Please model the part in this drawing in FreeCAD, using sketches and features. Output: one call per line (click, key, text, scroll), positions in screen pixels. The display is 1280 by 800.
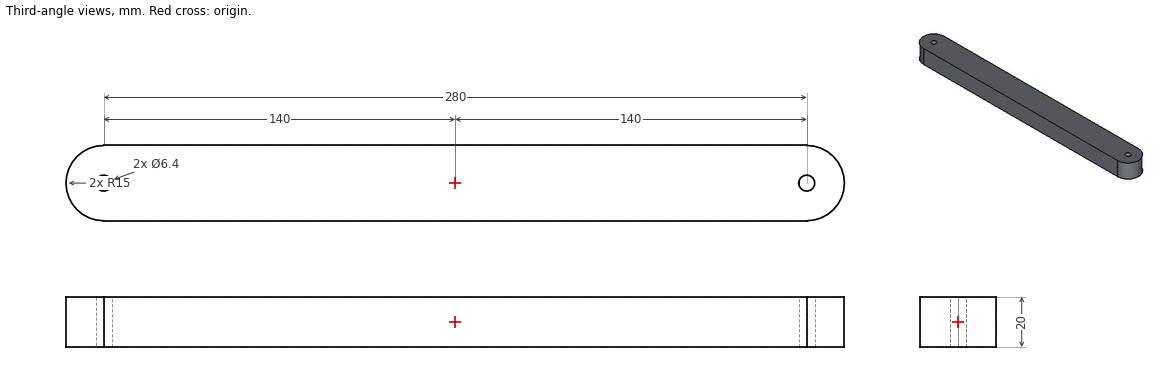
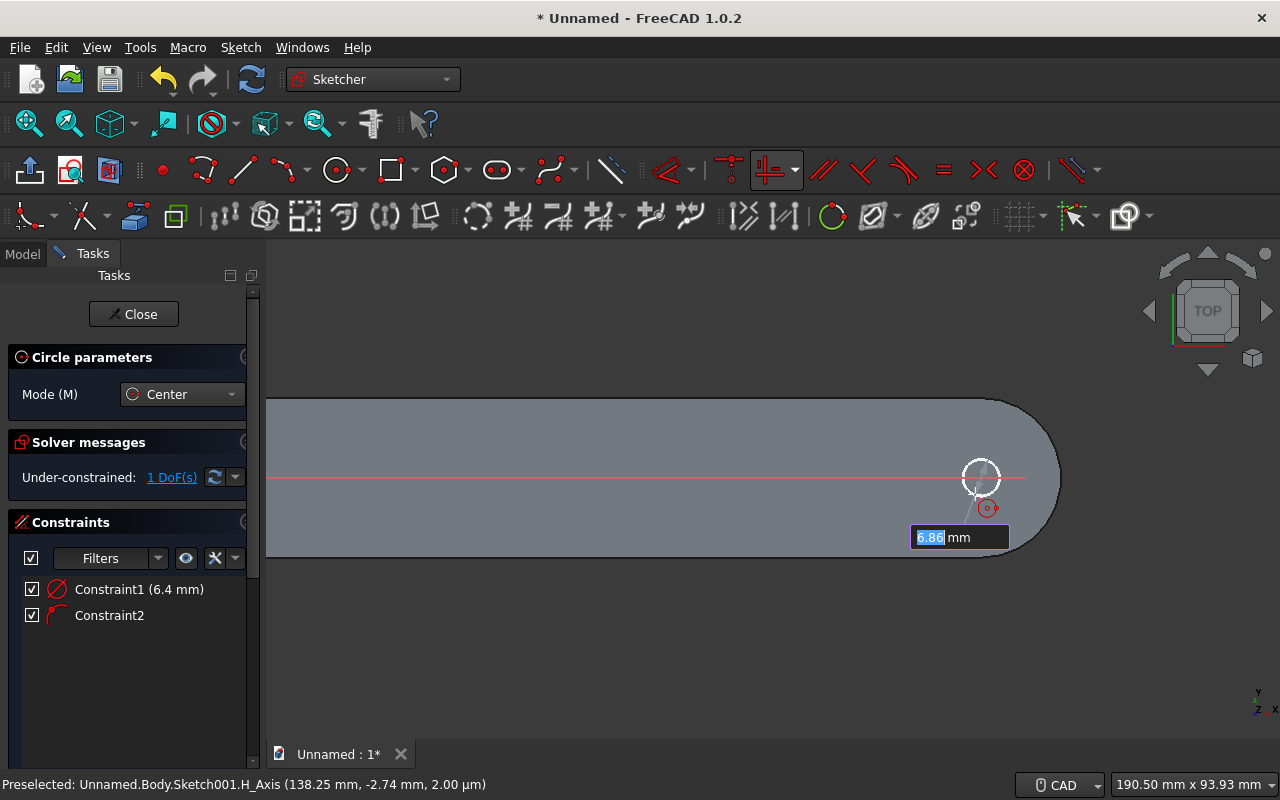
text(6.4)
key(Return)
key(Escape)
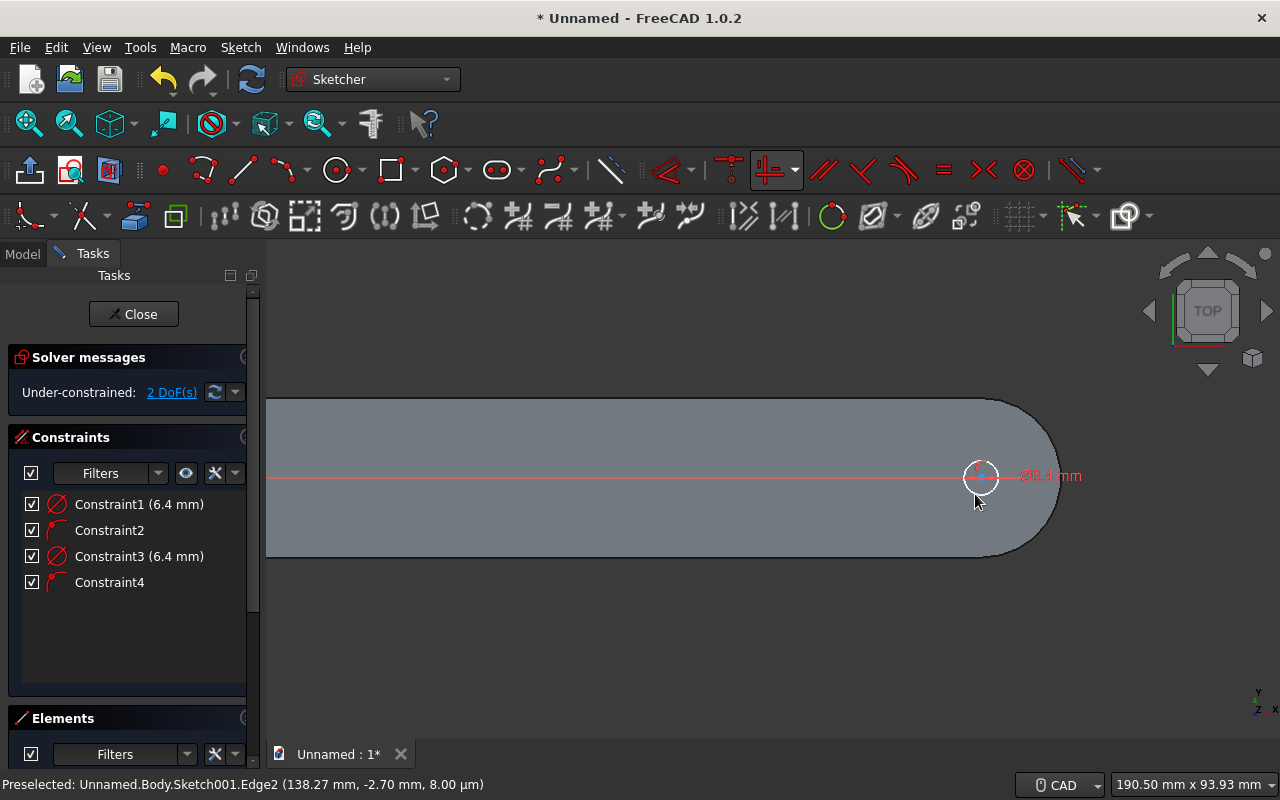
scroll(977, 495, down, 5)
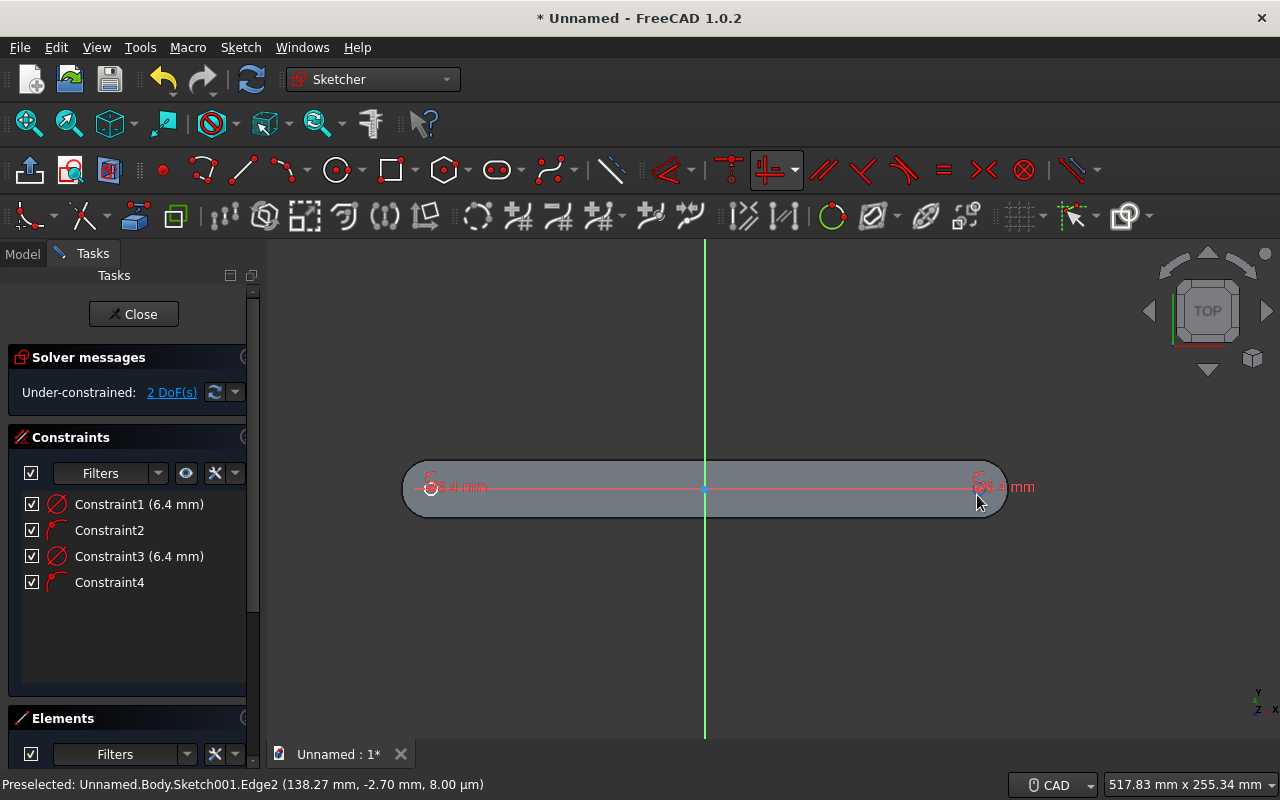
click(431, 489)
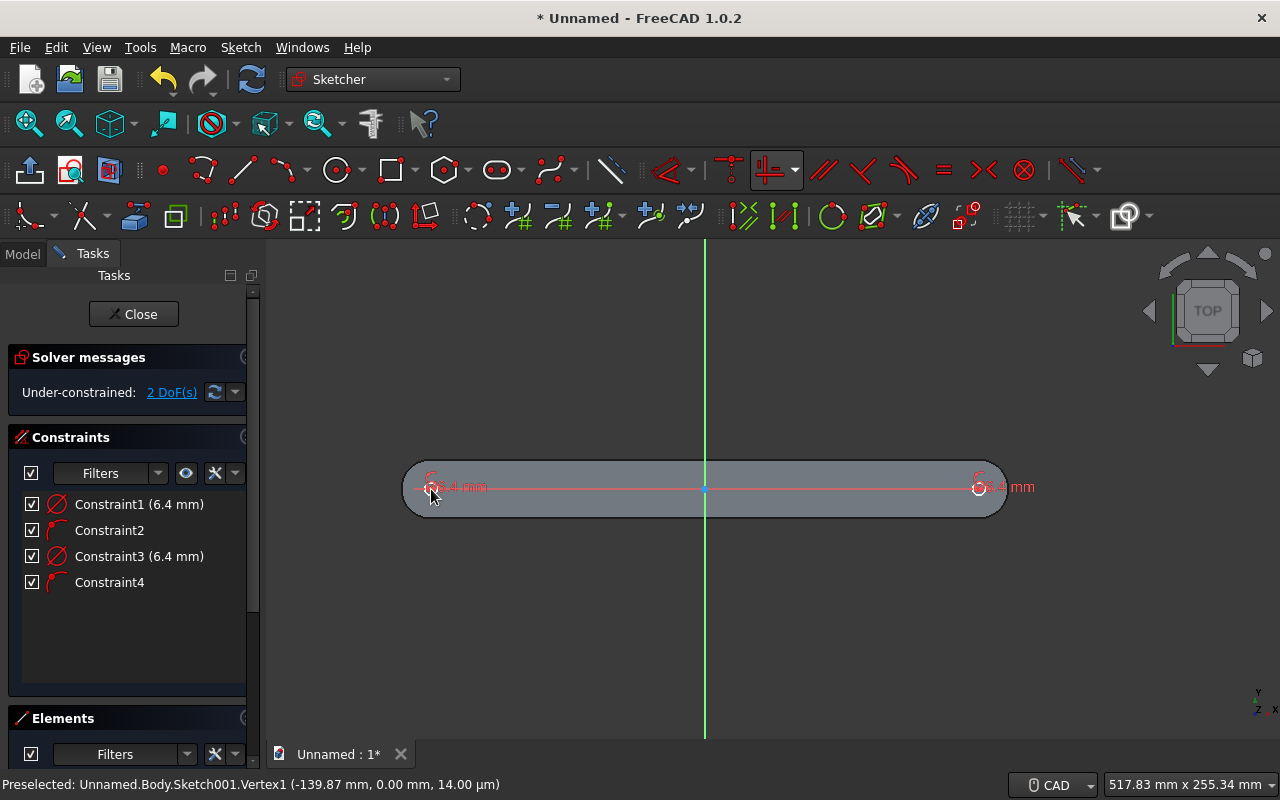
click(694, 170)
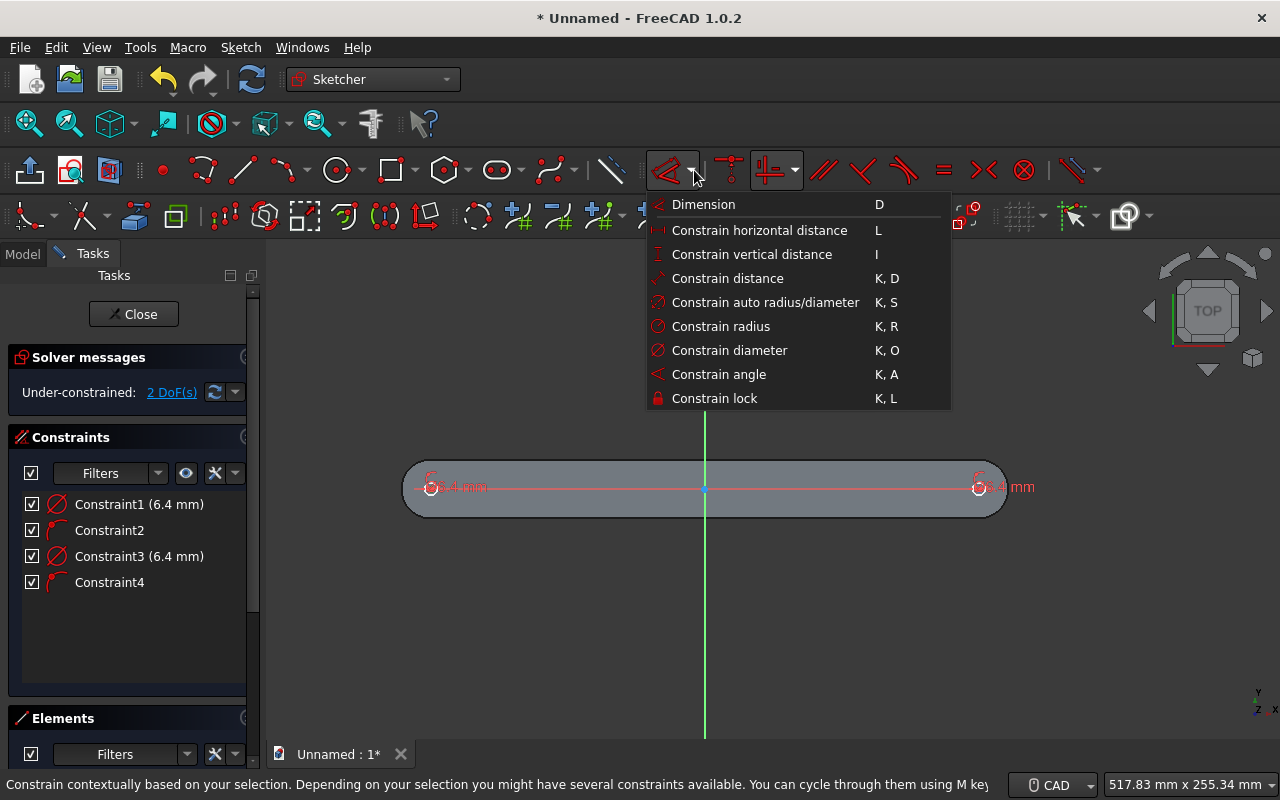
click(799, 230)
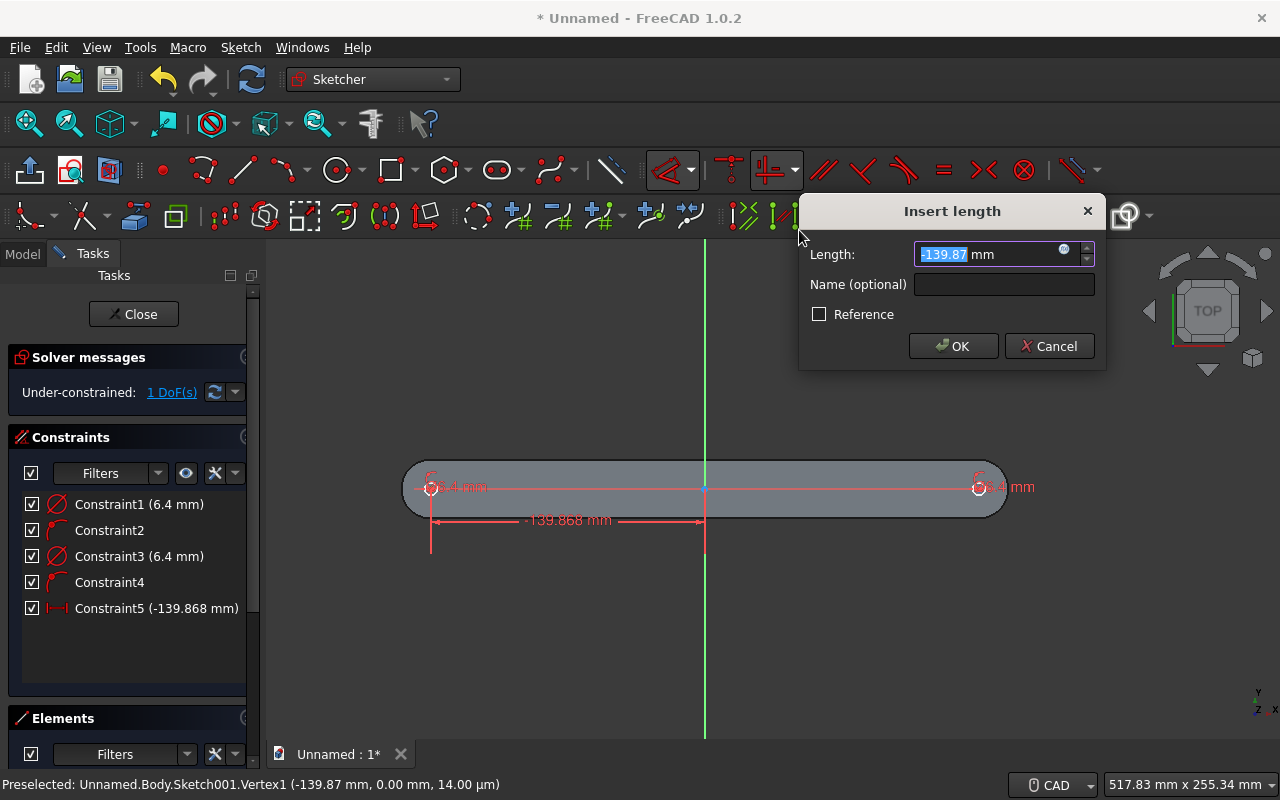
text(-140)
key(Return)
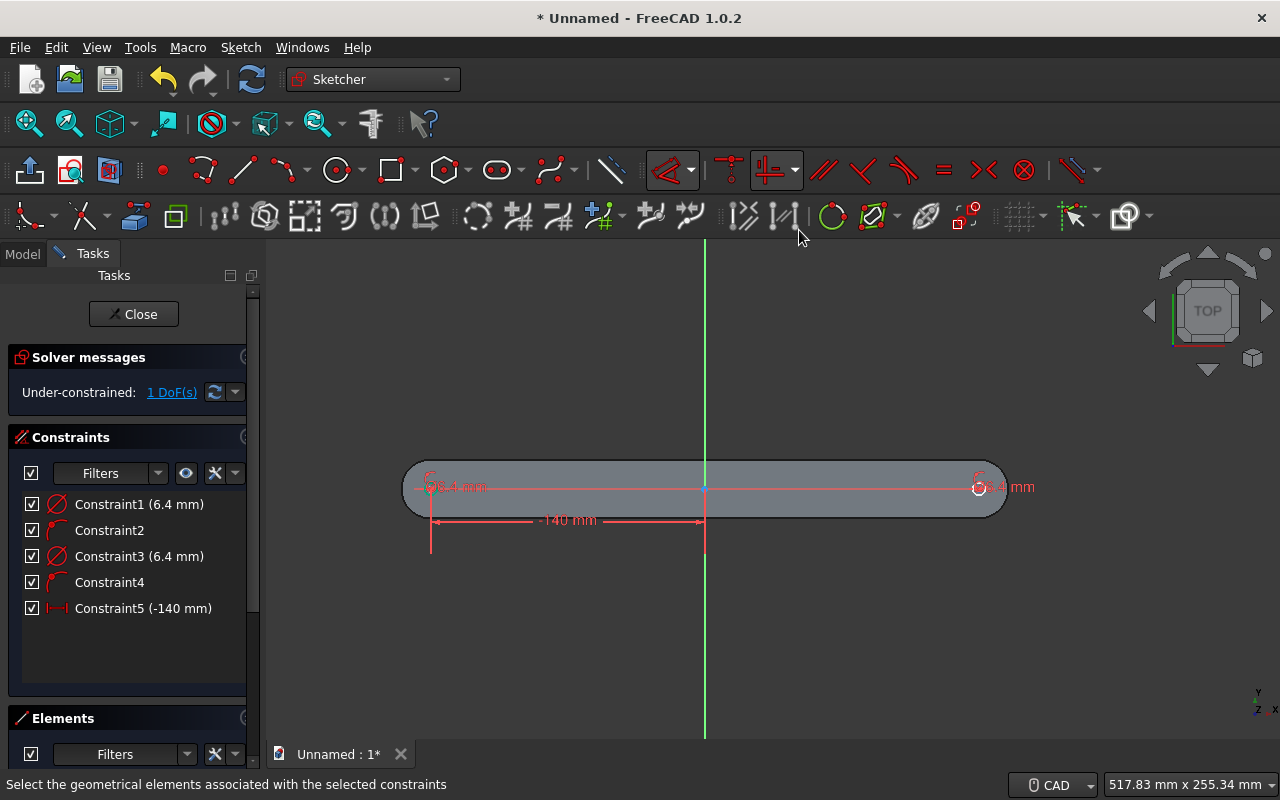
click(979, 489)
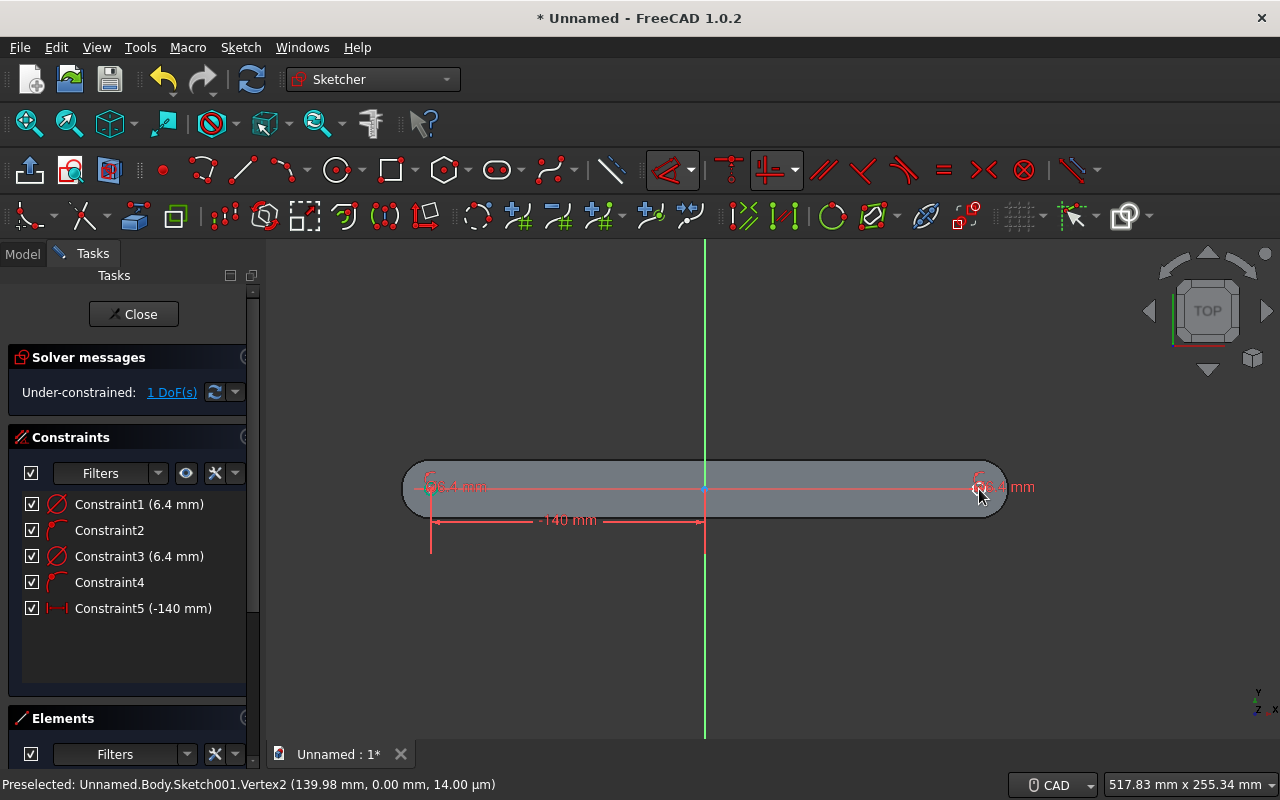
click(694, 170)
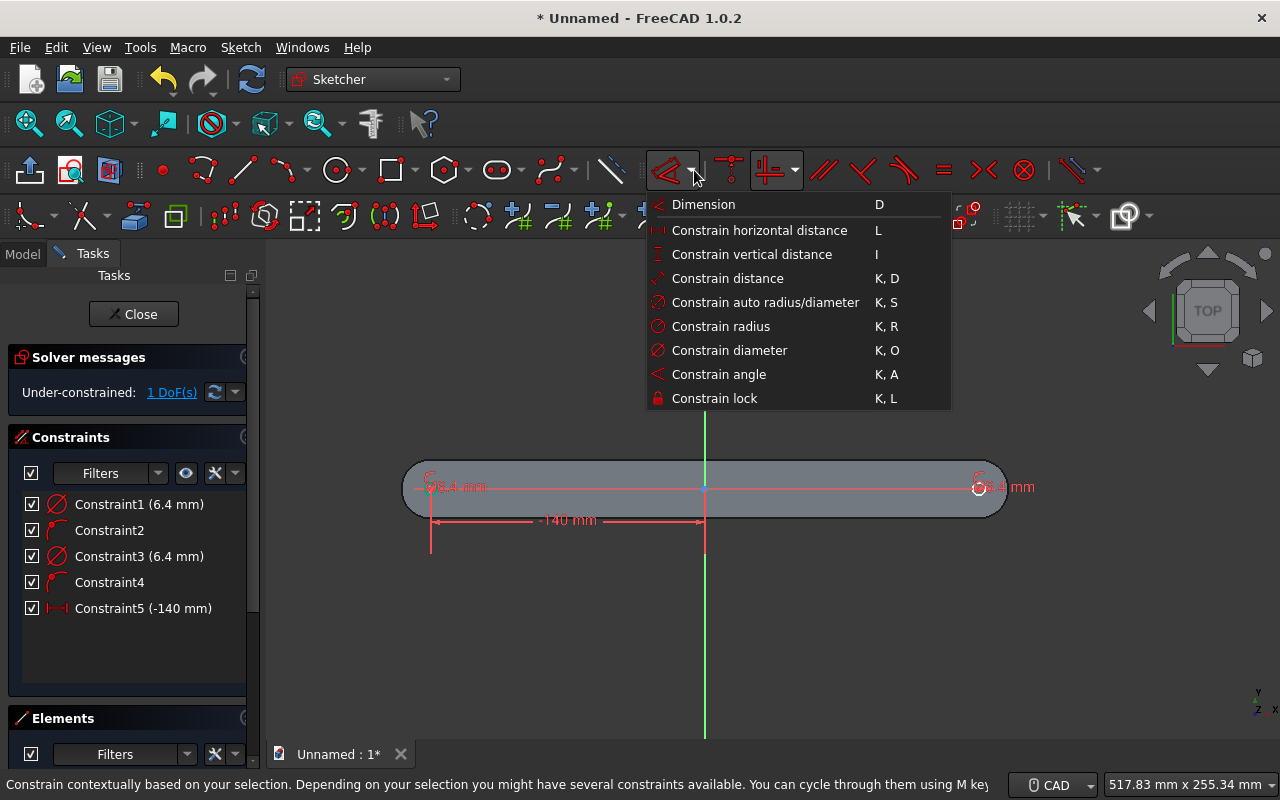
click(799, 230)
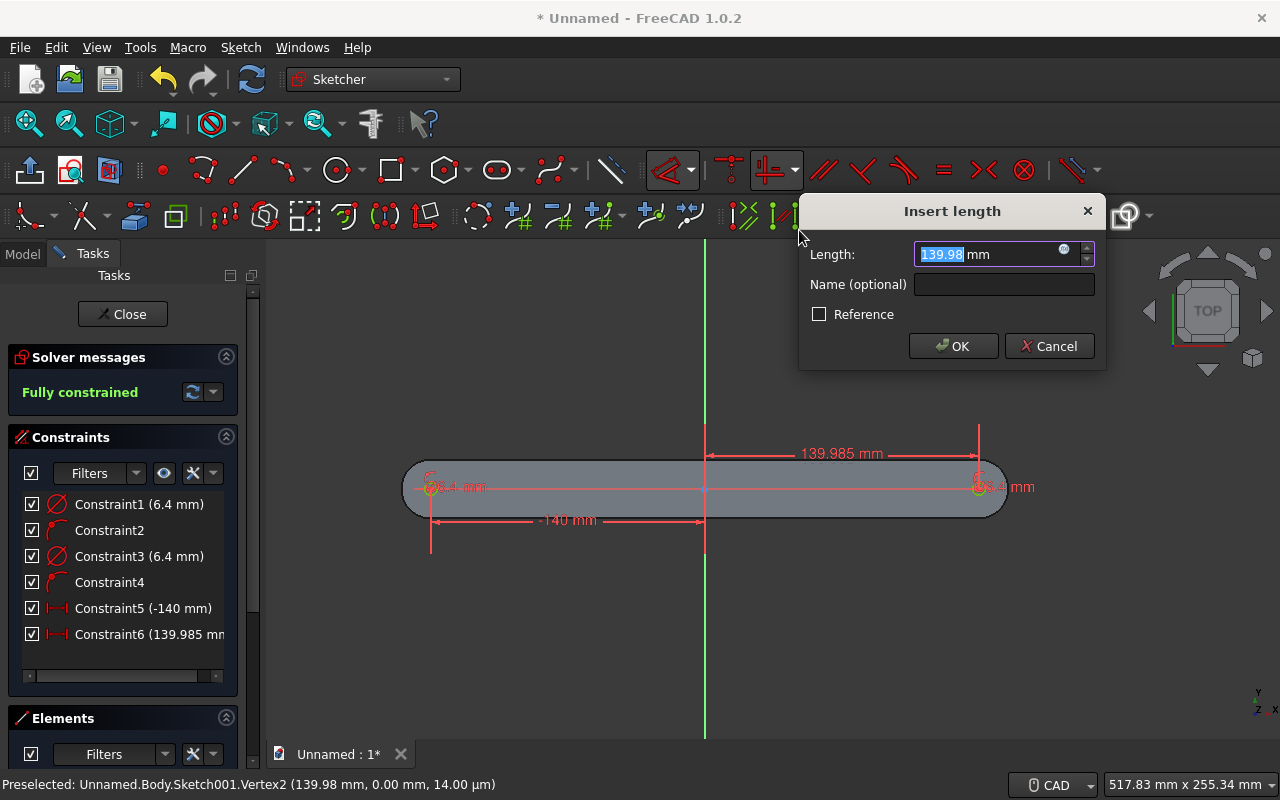
text(140)
key(Return)